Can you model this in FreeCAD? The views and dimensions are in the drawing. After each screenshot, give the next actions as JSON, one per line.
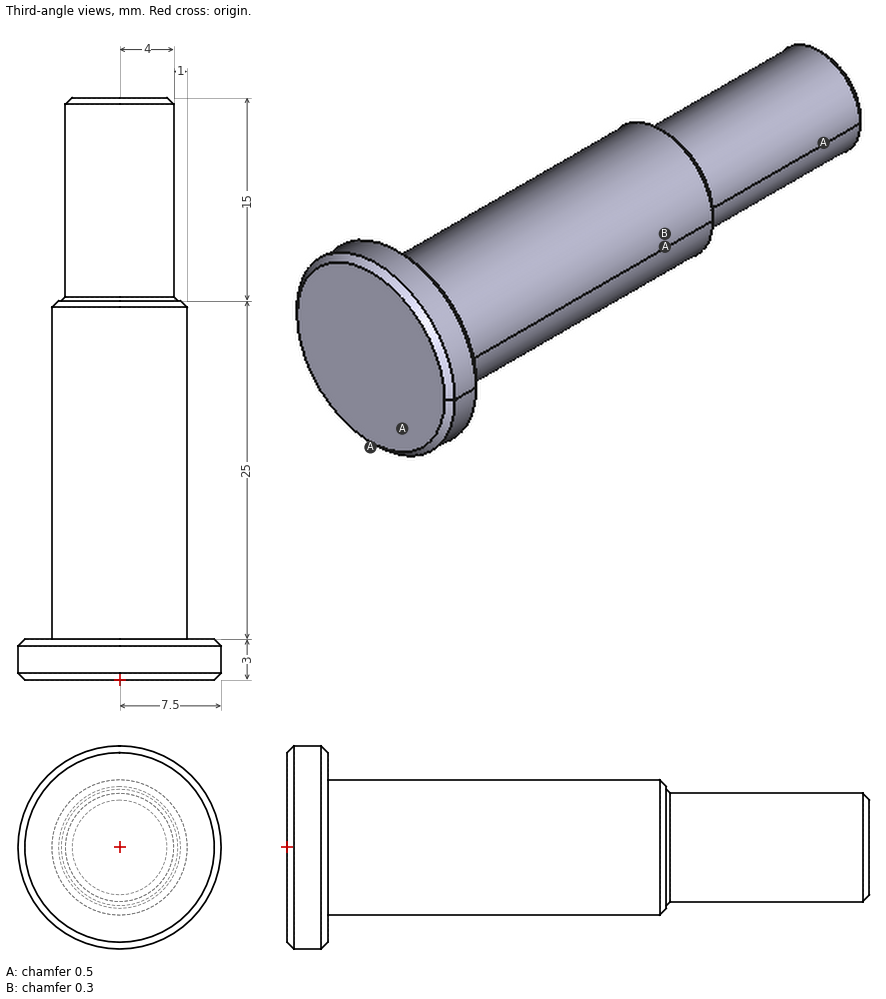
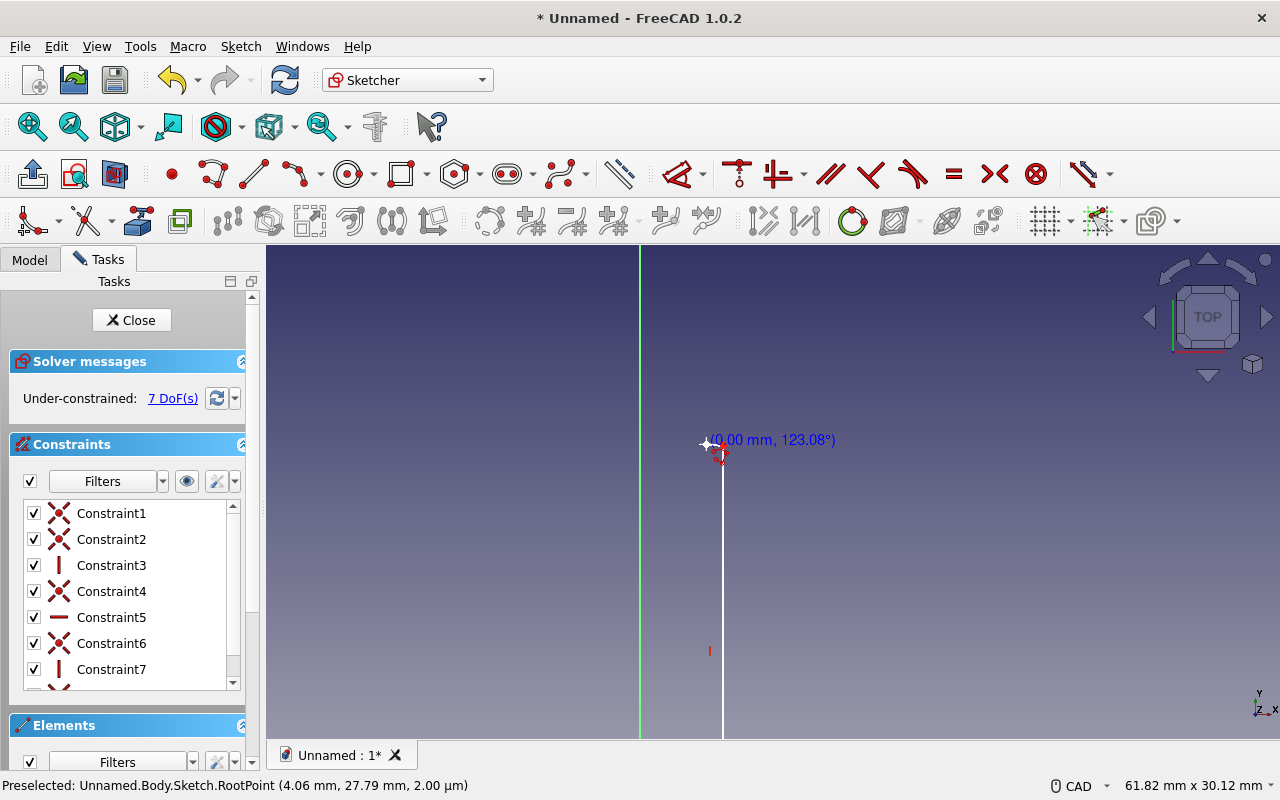
{"action": "scroll", "coordinate": [707, 445], "scroll_direction": "down", "scroll_amount": 4}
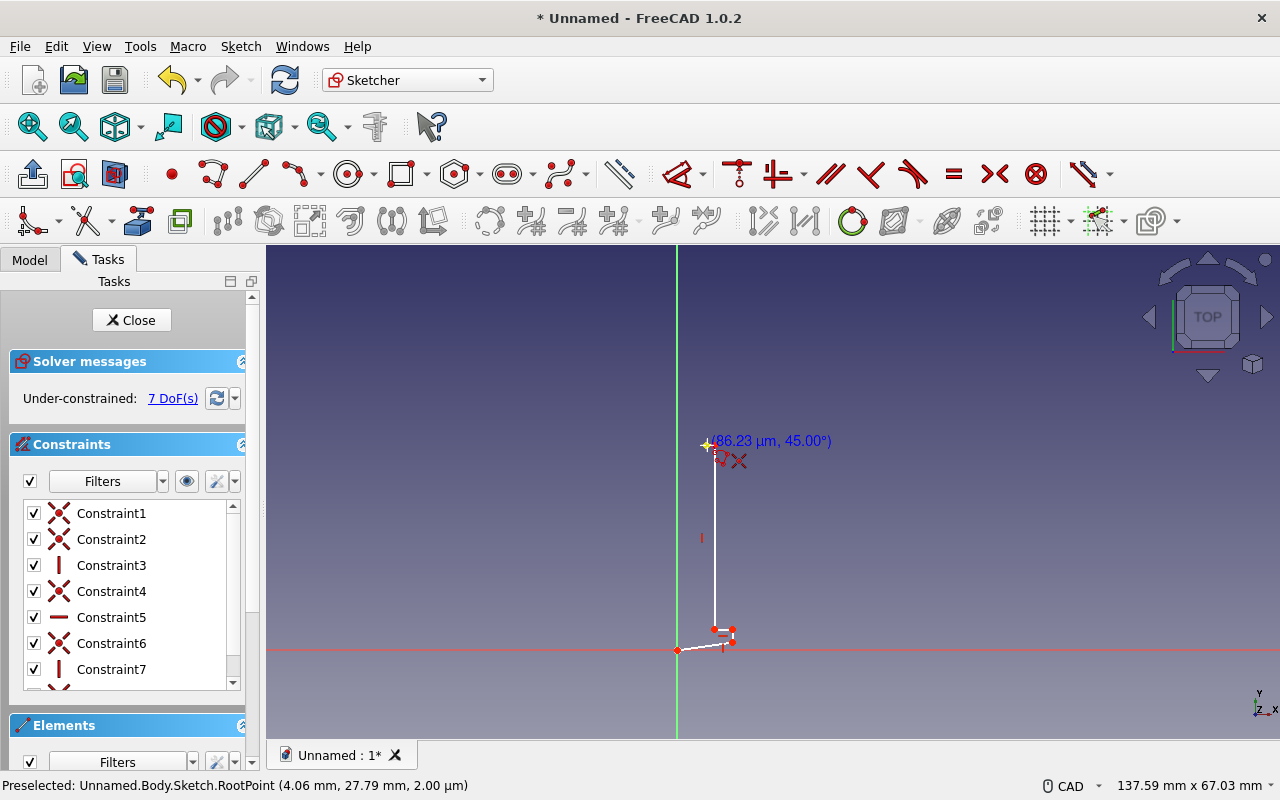
{"action": "left_click", "coordinate": [707, 334]}
{"action": "left_click", "coordinate": [686, 334]}
{"action": "left_click", "coordinate": [677, 650]}
{"action": "key", "text": "Escape"}
{"action": "key", "text": "Escape"}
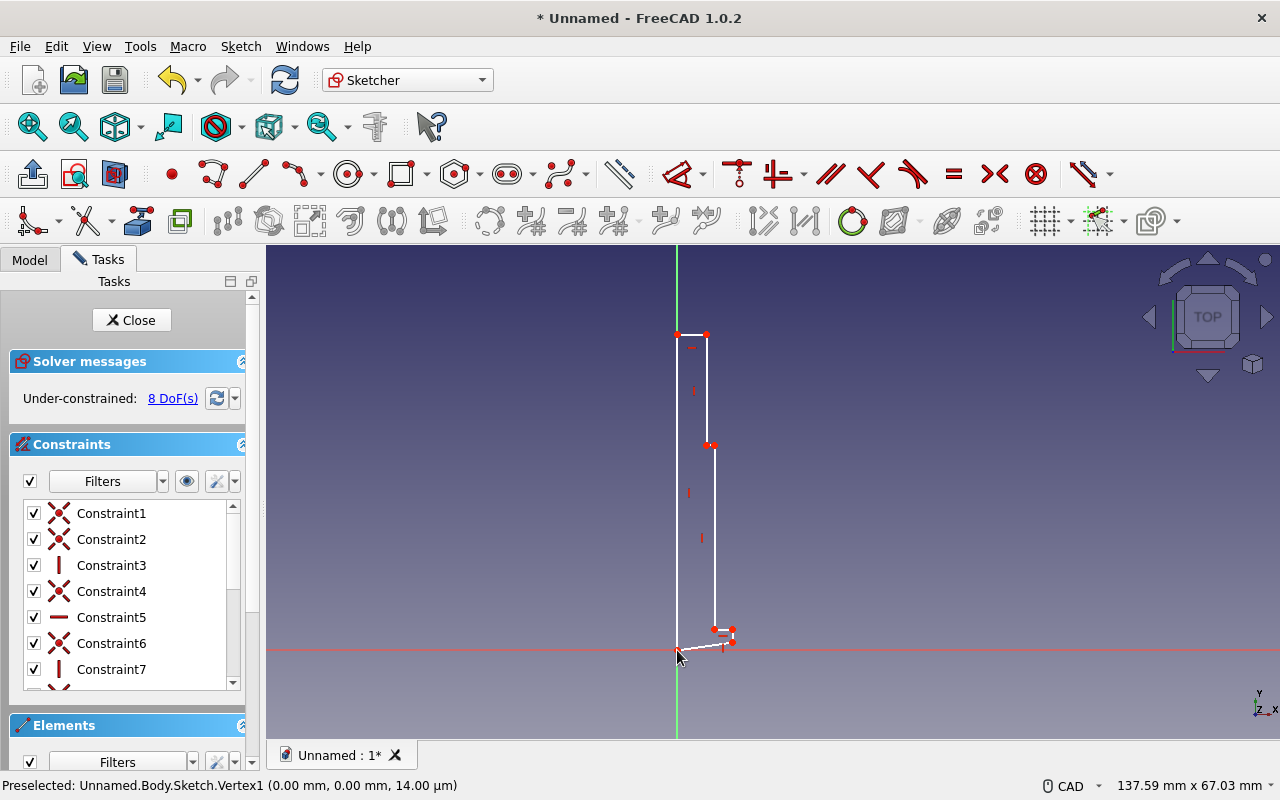
{"action": "left_click", "coordinate": [694, 648]}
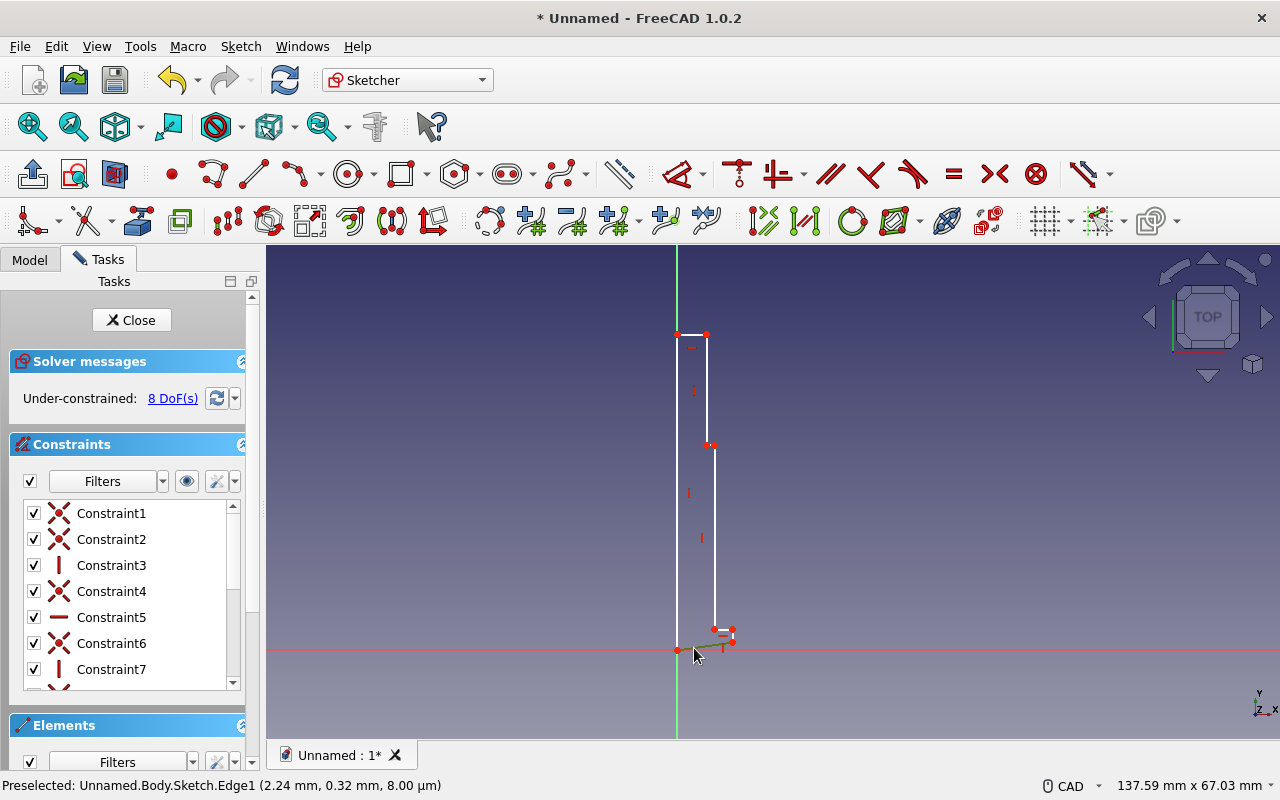
{"action": "key", "text": "h"}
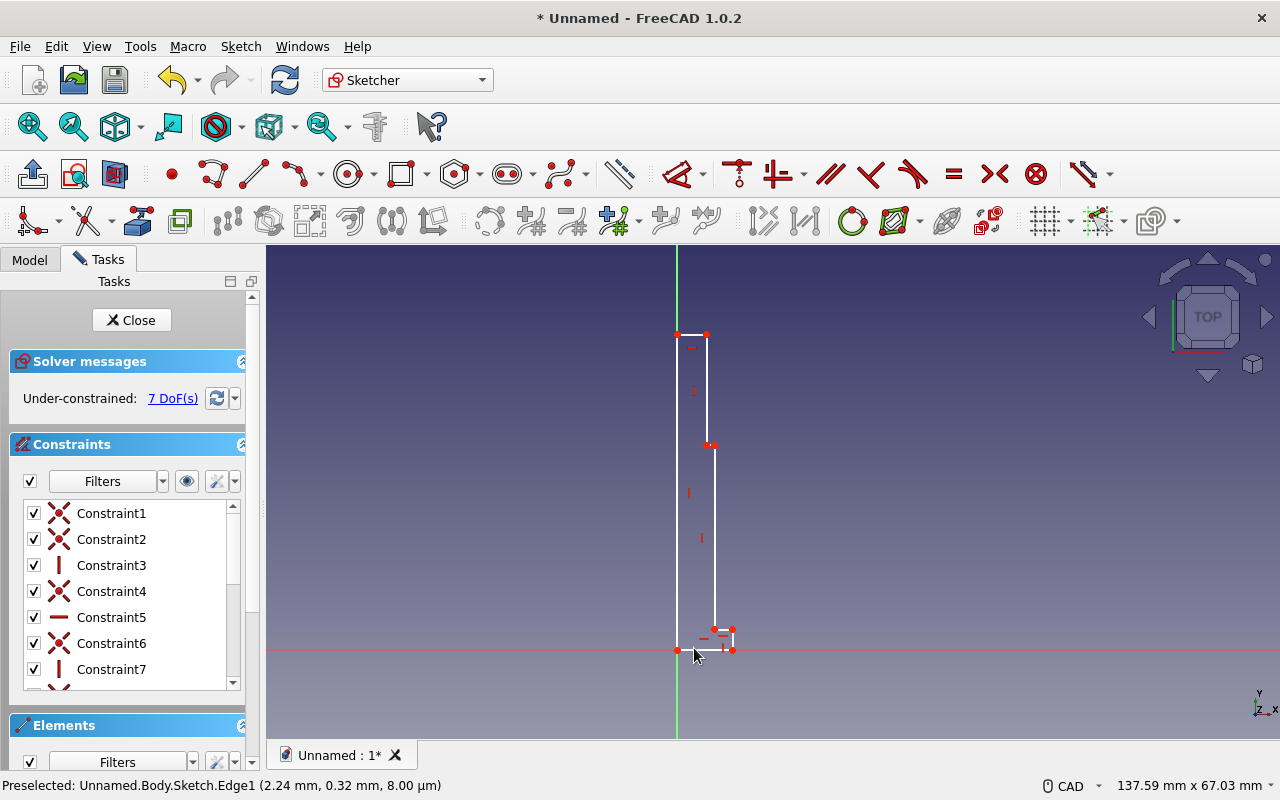
{"action": "scroll", "coordinate": [711, 445], "scroll_direction": "up", "scroll_amount": 7}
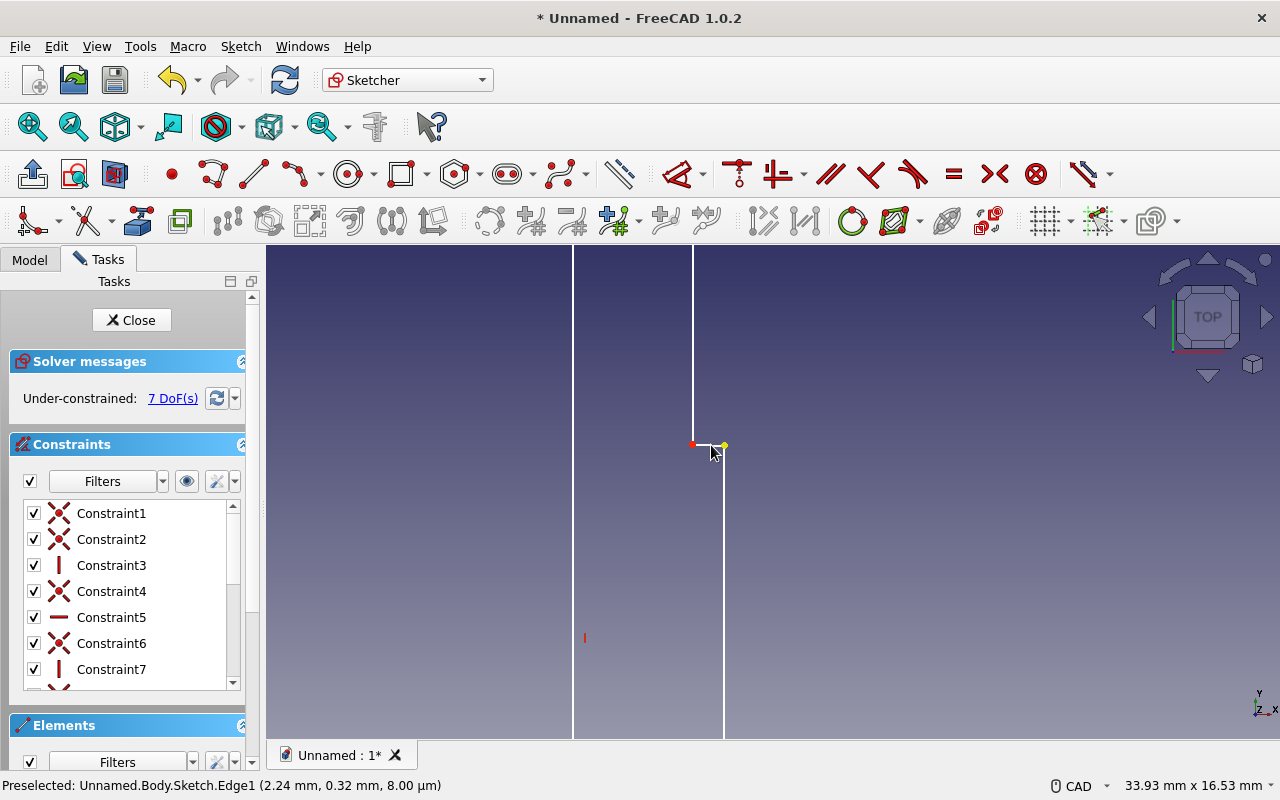
{"action": "left_click", "coordinate": [708, 445]}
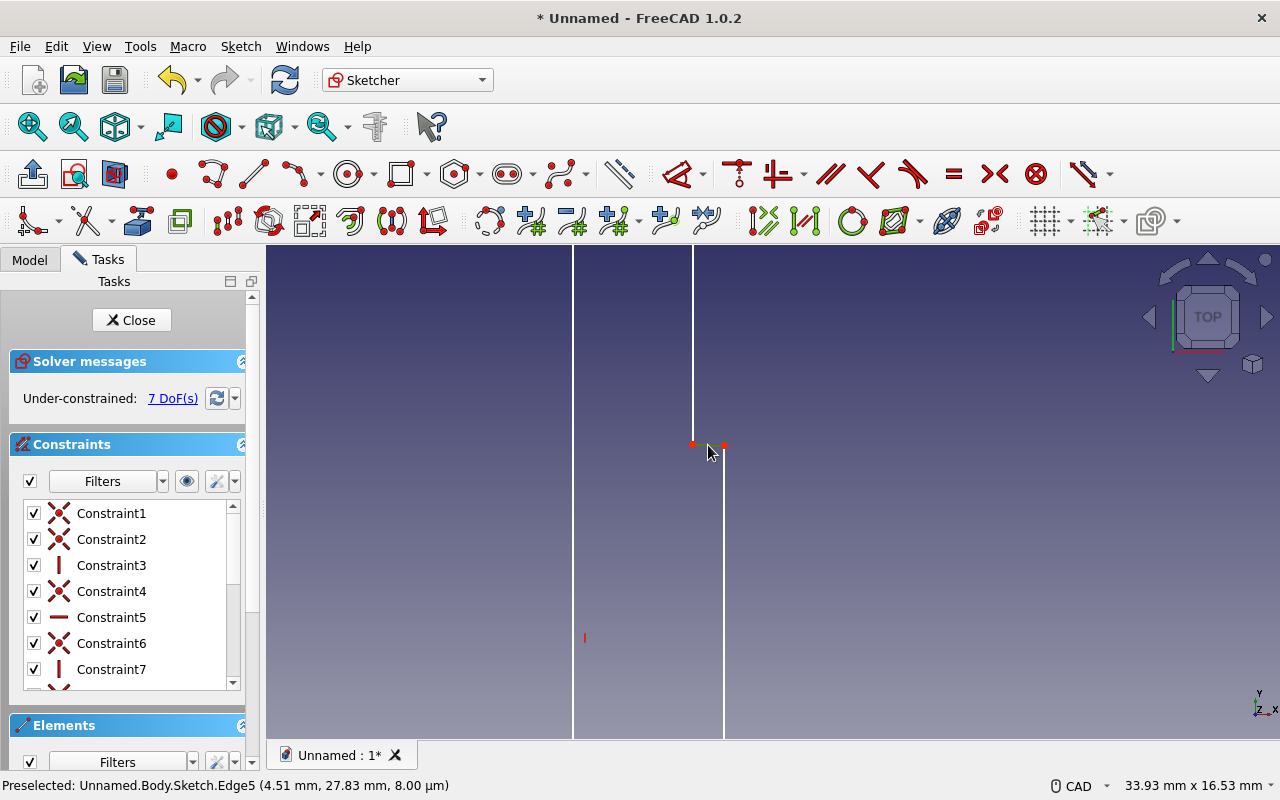
{"action": "left_click", "coordinate": [804, 174]}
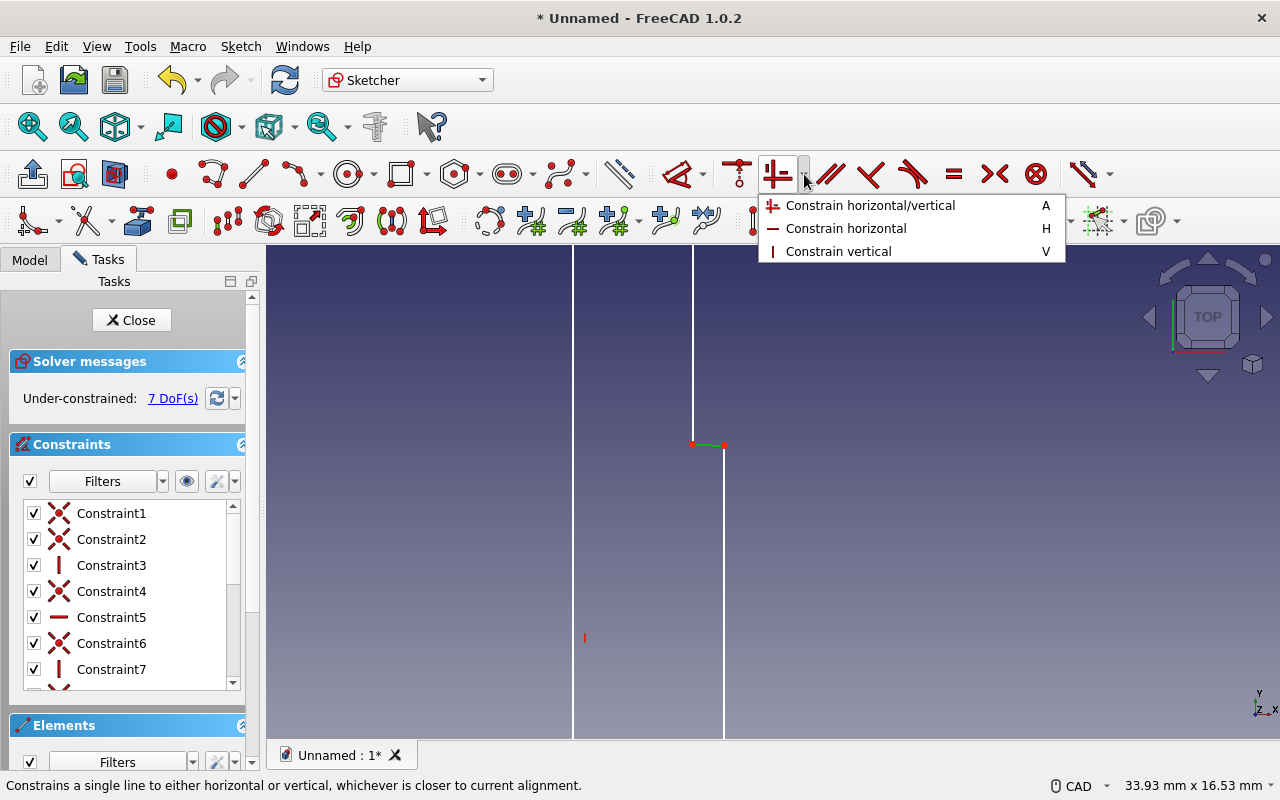
{"action": "left_click", "coordinate": [912, 228]}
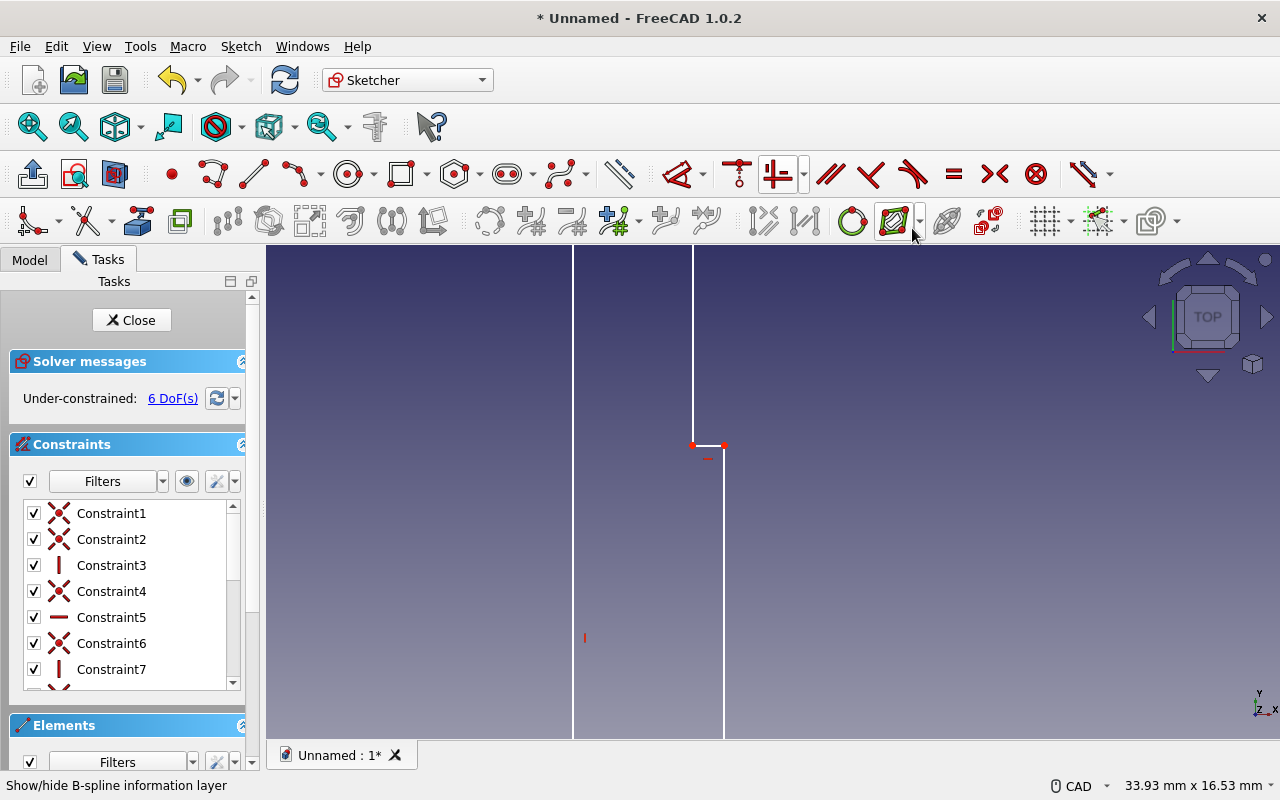
{"action": "left_click", "coordinate": [676, 174]}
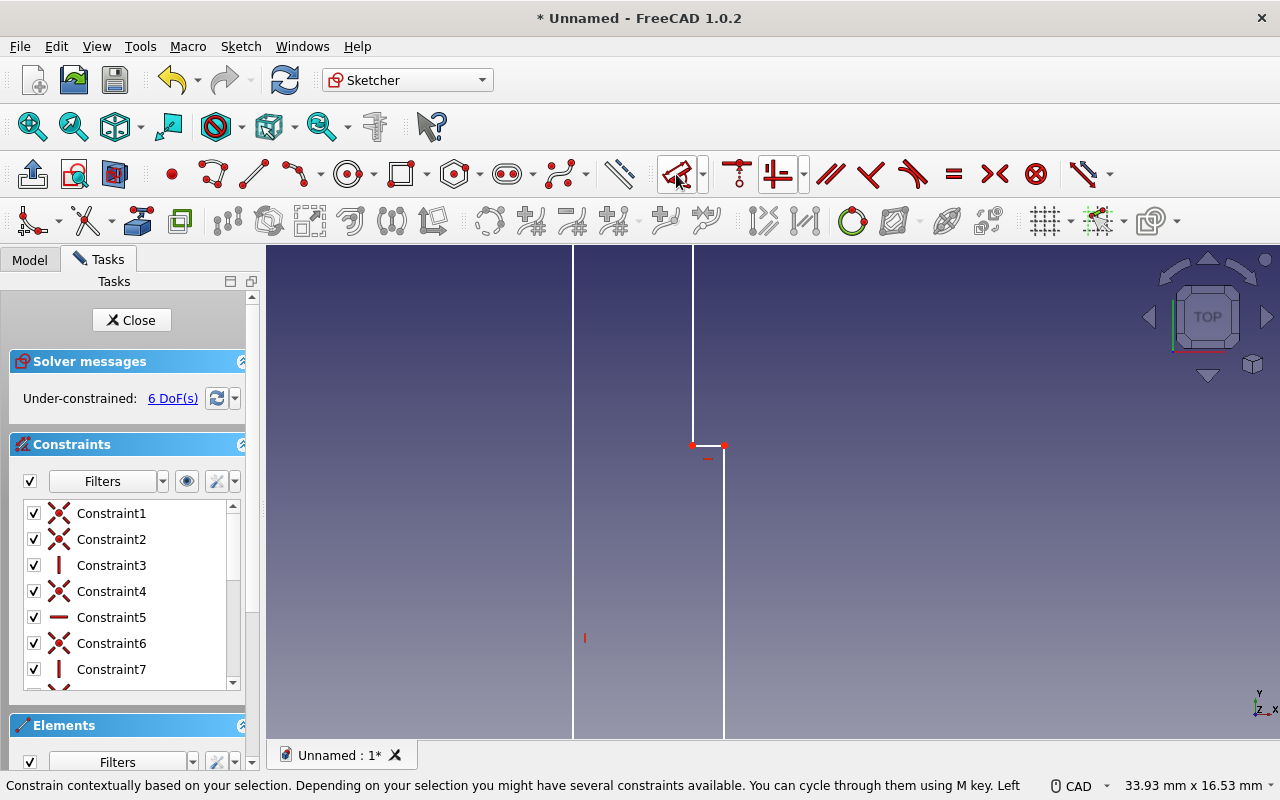
{"action": "scroll", "coordinate": [711, 445], "scroll_direction": "down", "scroll_amount": 7}